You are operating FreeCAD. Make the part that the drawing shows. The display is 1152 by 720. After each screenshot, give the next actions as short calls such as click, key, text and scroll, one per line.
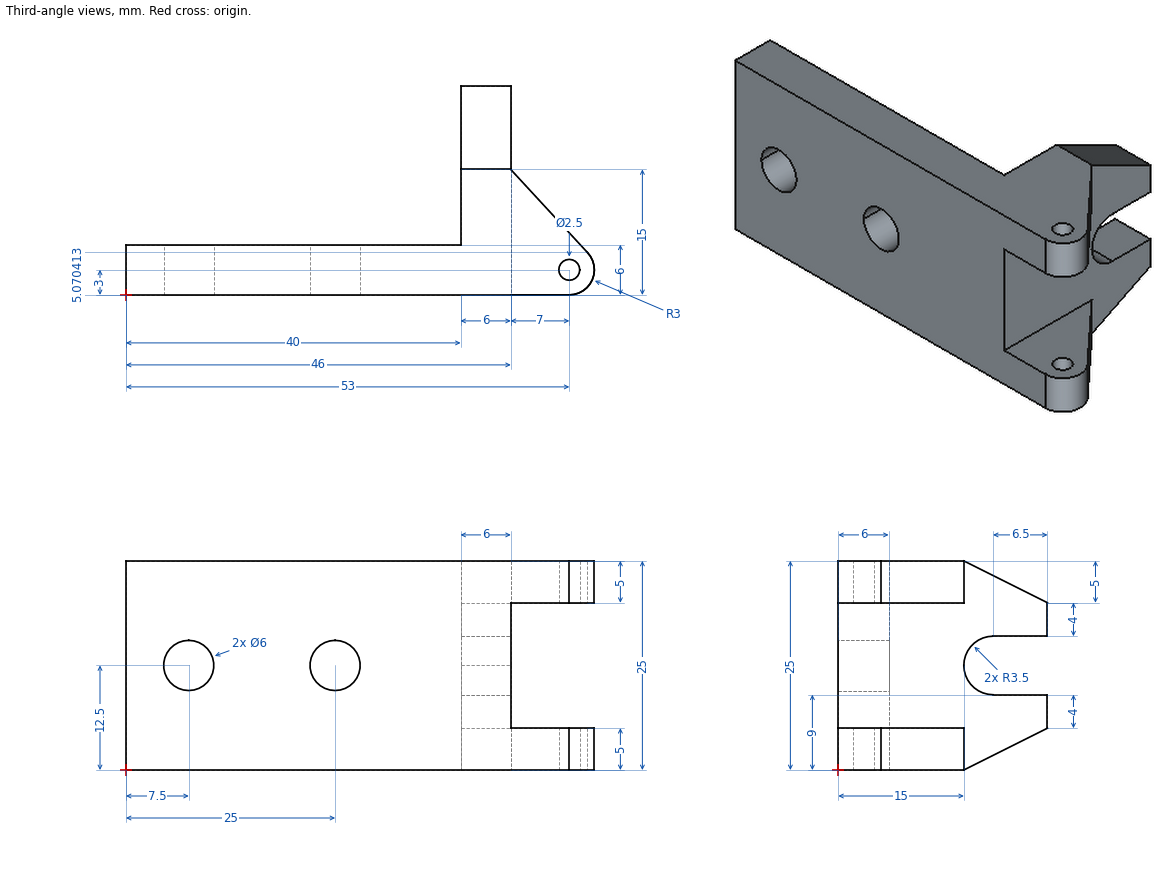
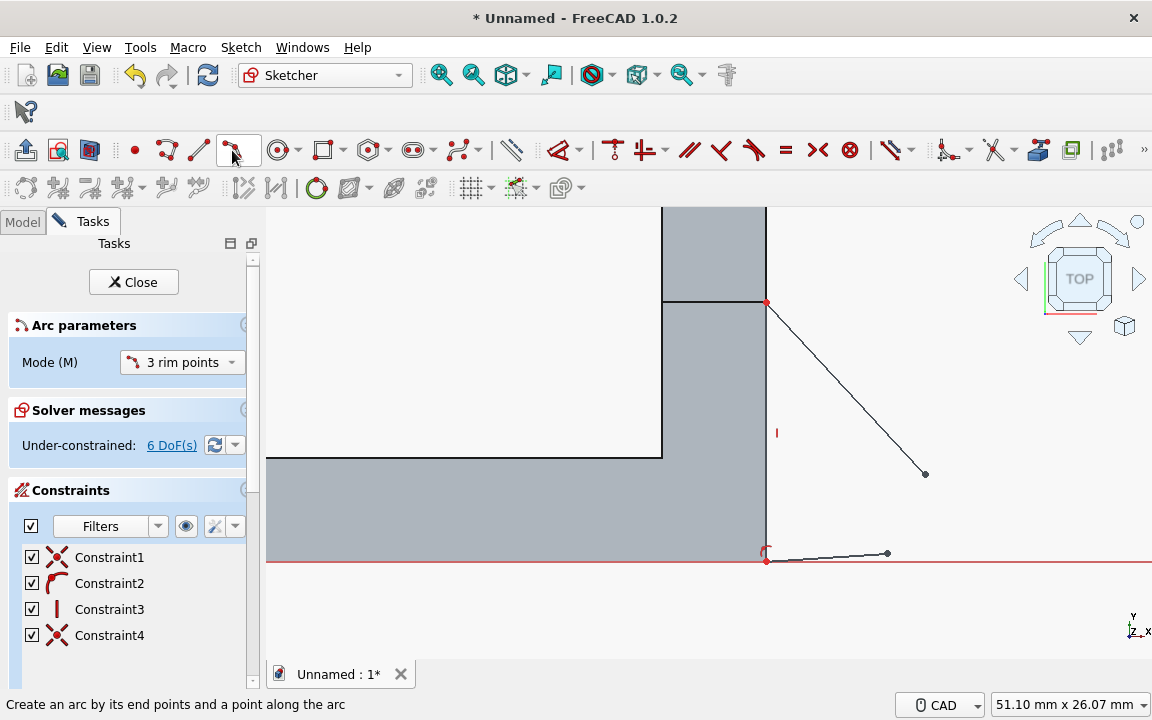
click(887, 554)
click(925, 475)
click(935, 530)
key(Escape)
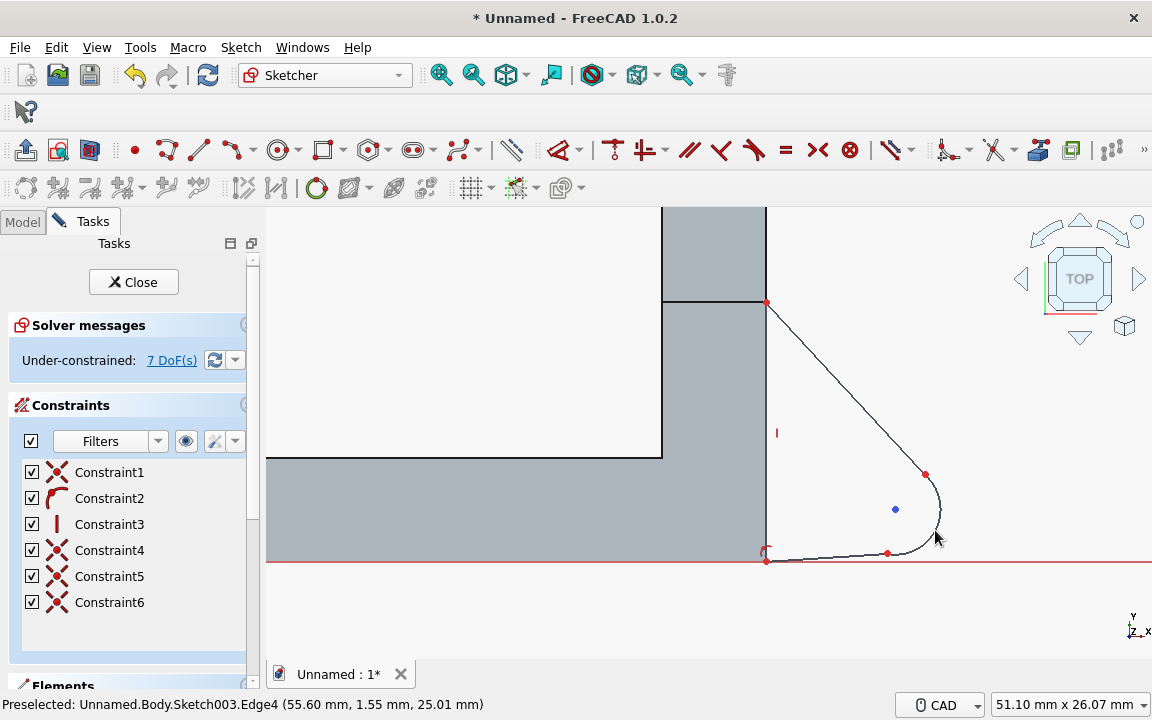
click(802, 560)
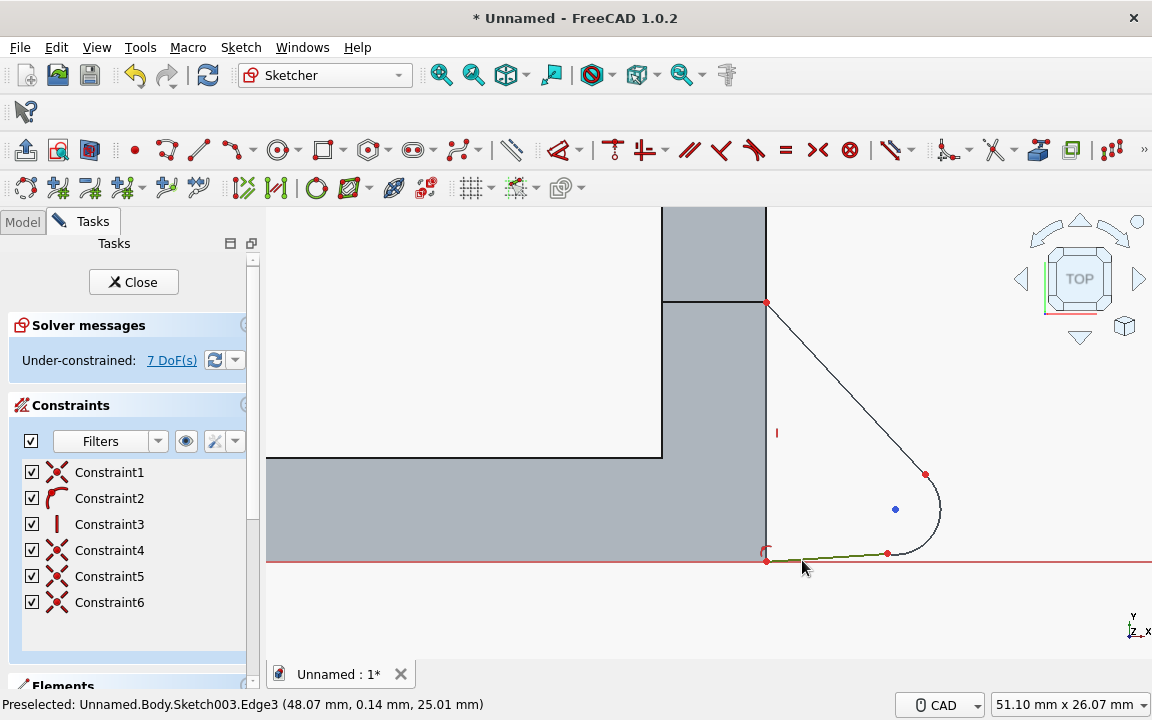
click(921, 547)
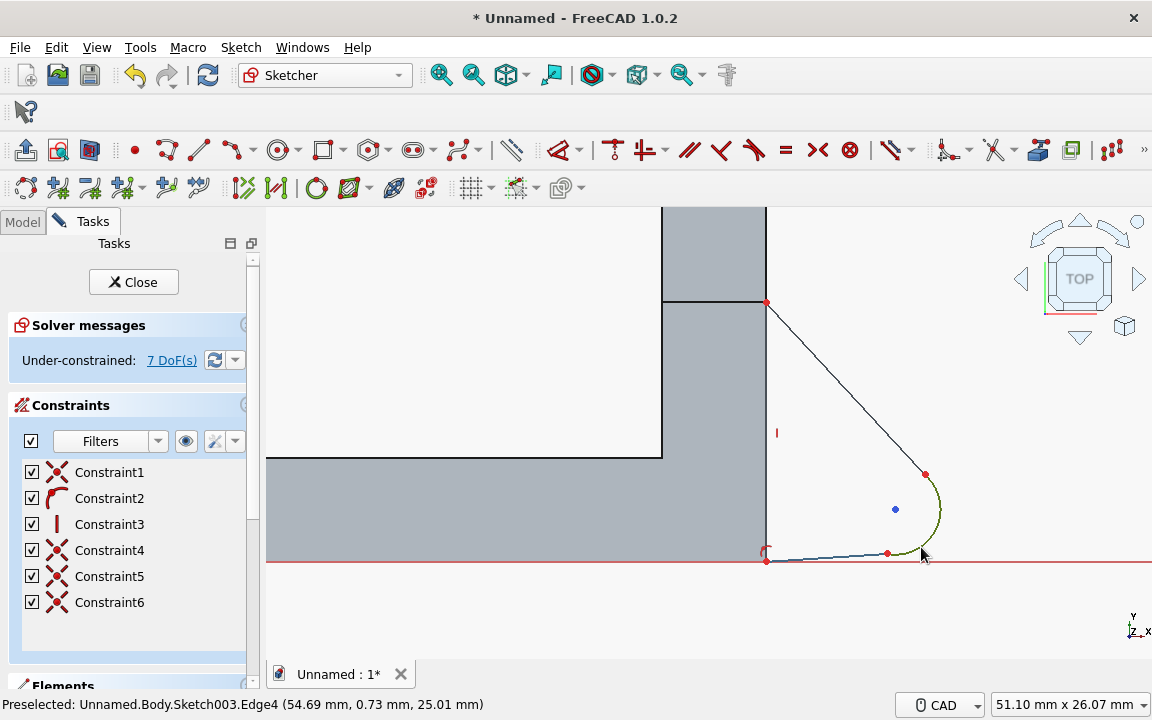
key(t)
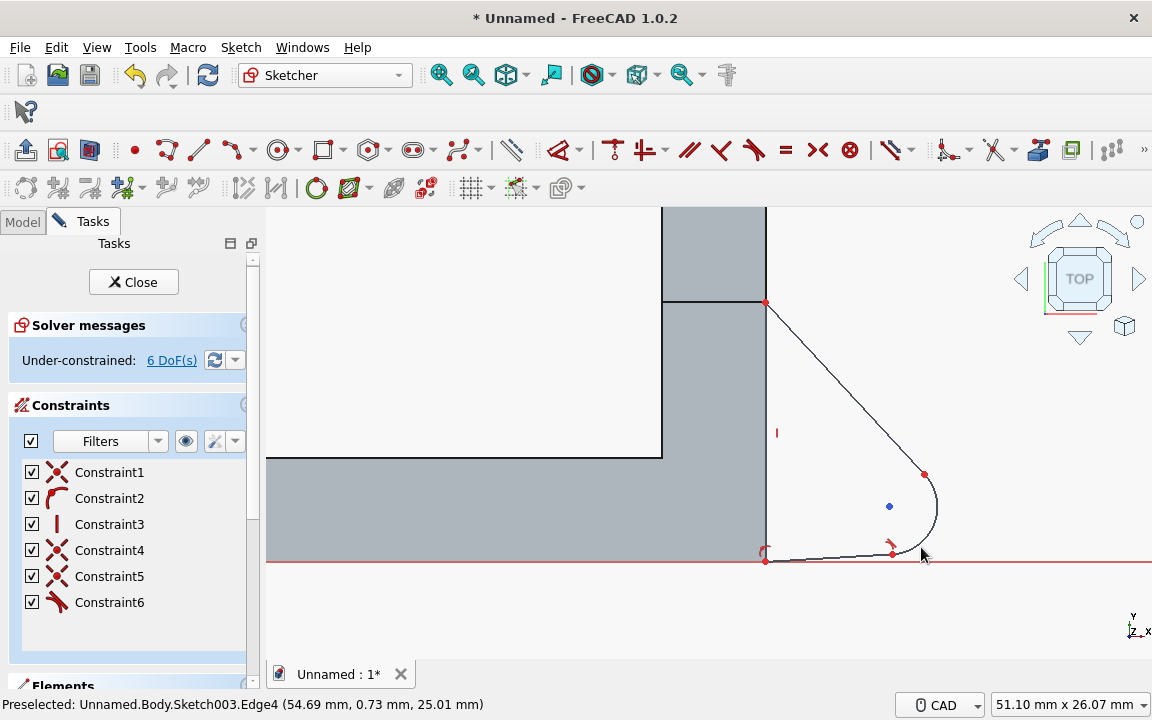
click(804, 560)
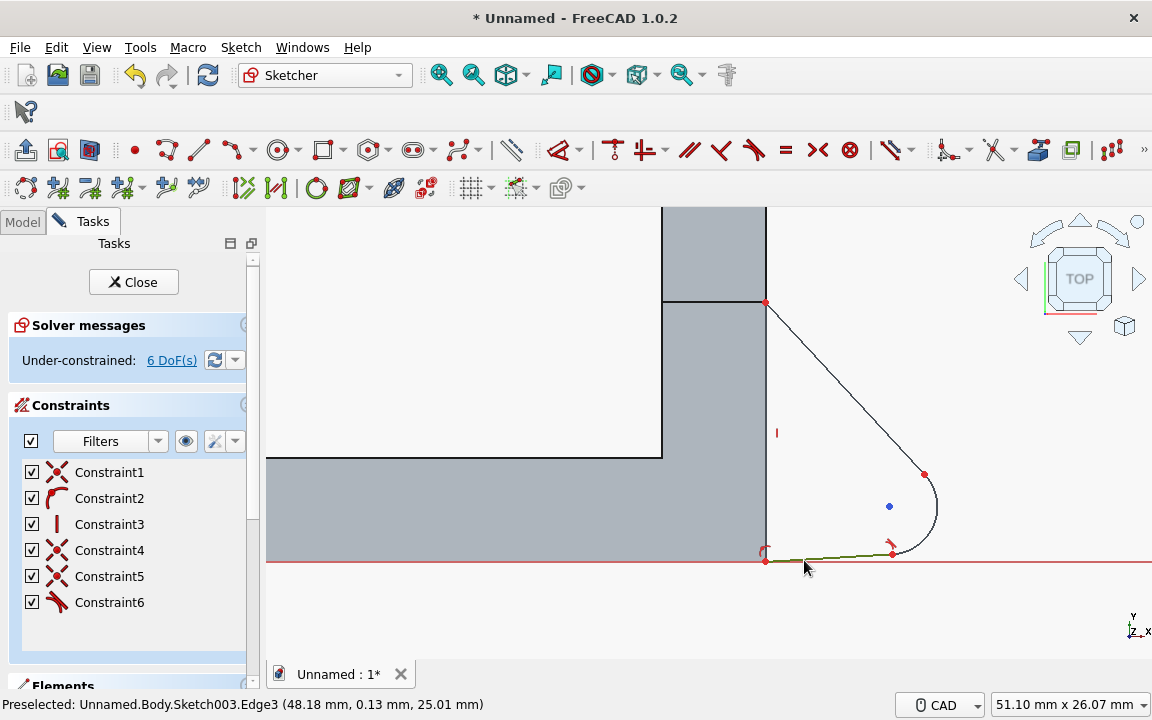
key(h)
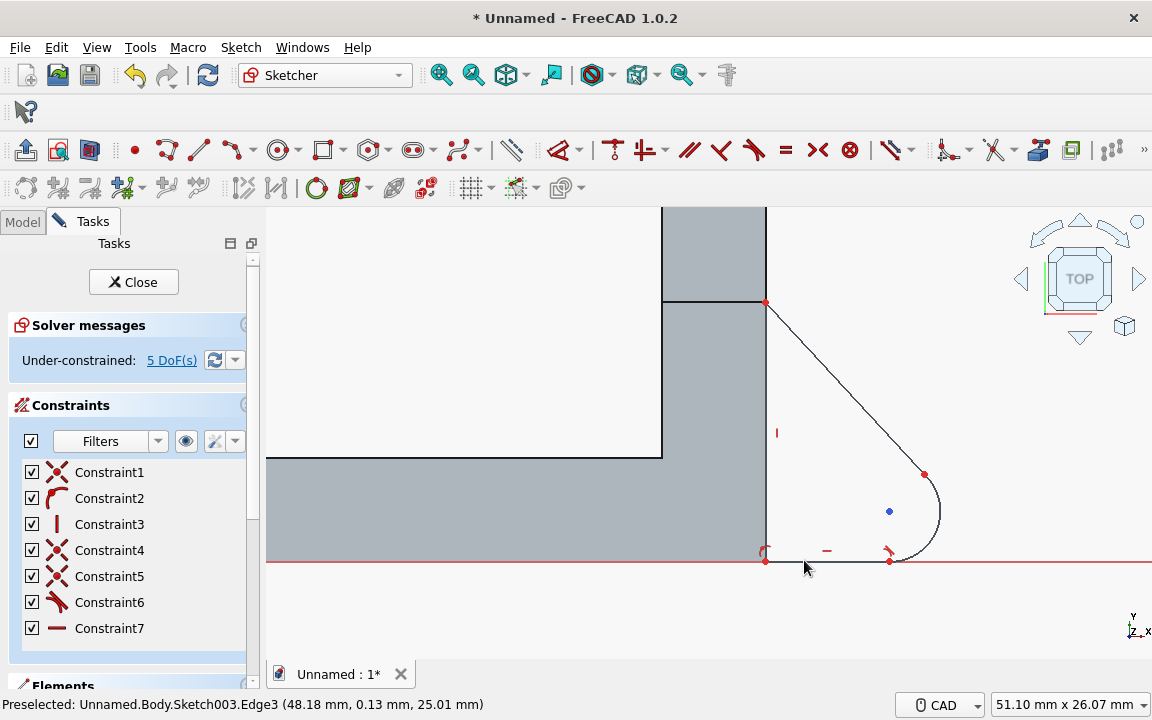
click(558, 150)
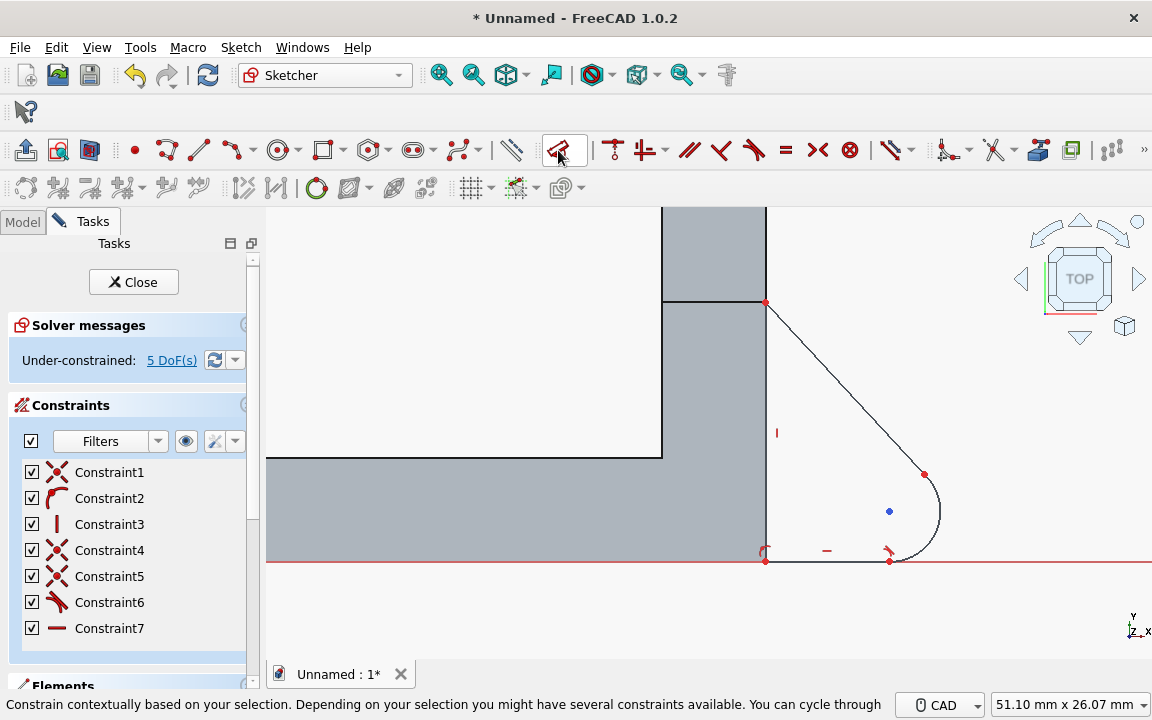
click(923, 550)
click(907, 592)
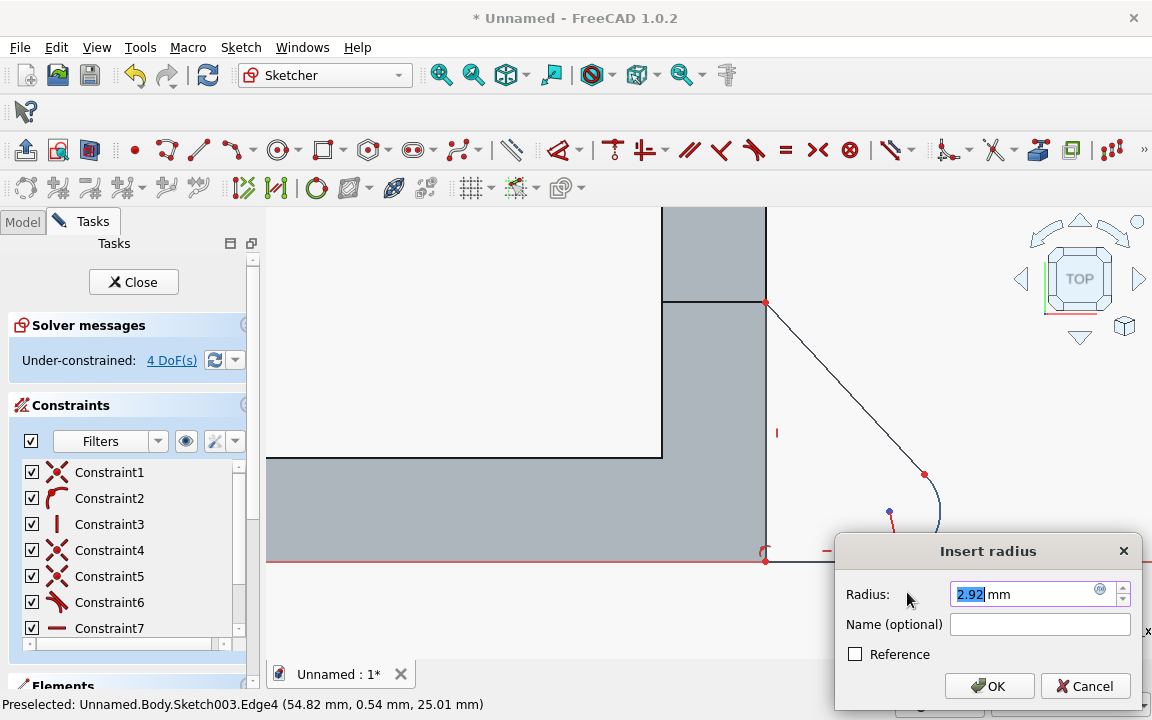
text(3)
key(Return)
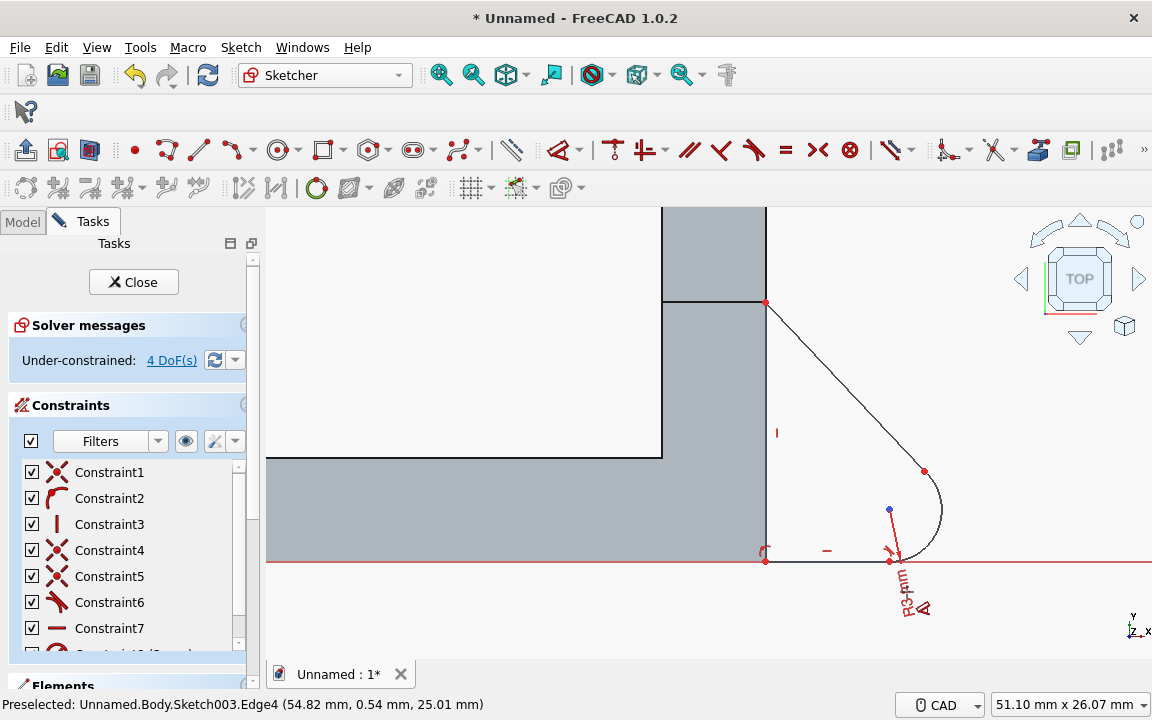
click(803, 562)
click(828, 596)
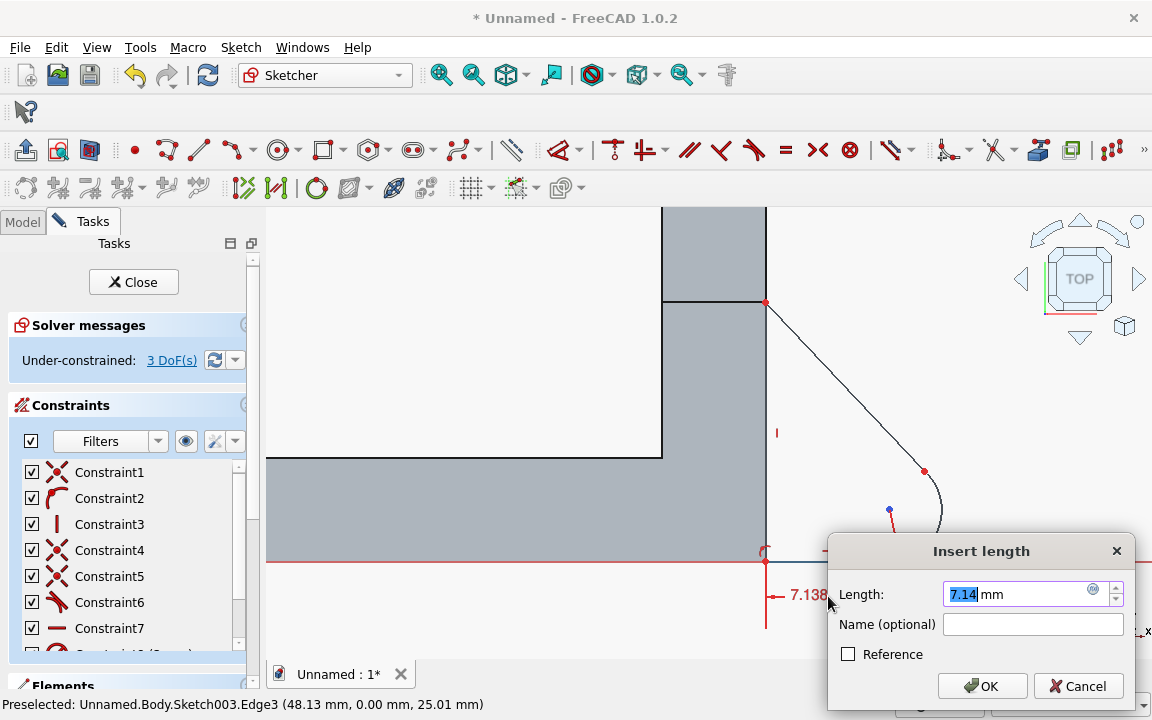
text(7)
key(Return)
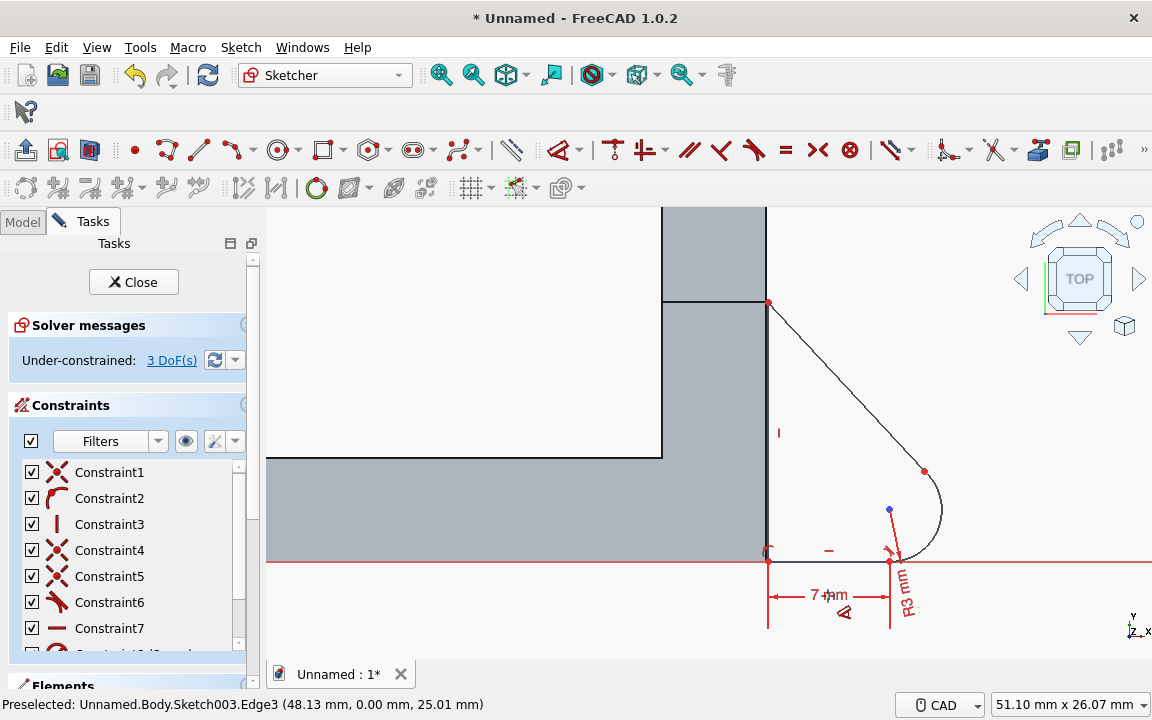
click(768, 381)
click(734, 432)